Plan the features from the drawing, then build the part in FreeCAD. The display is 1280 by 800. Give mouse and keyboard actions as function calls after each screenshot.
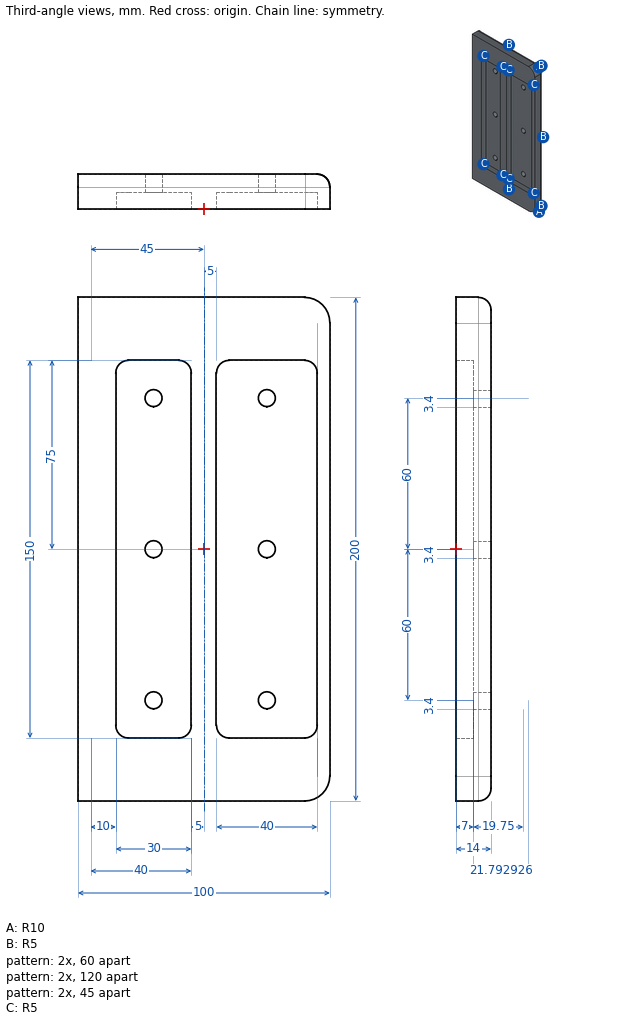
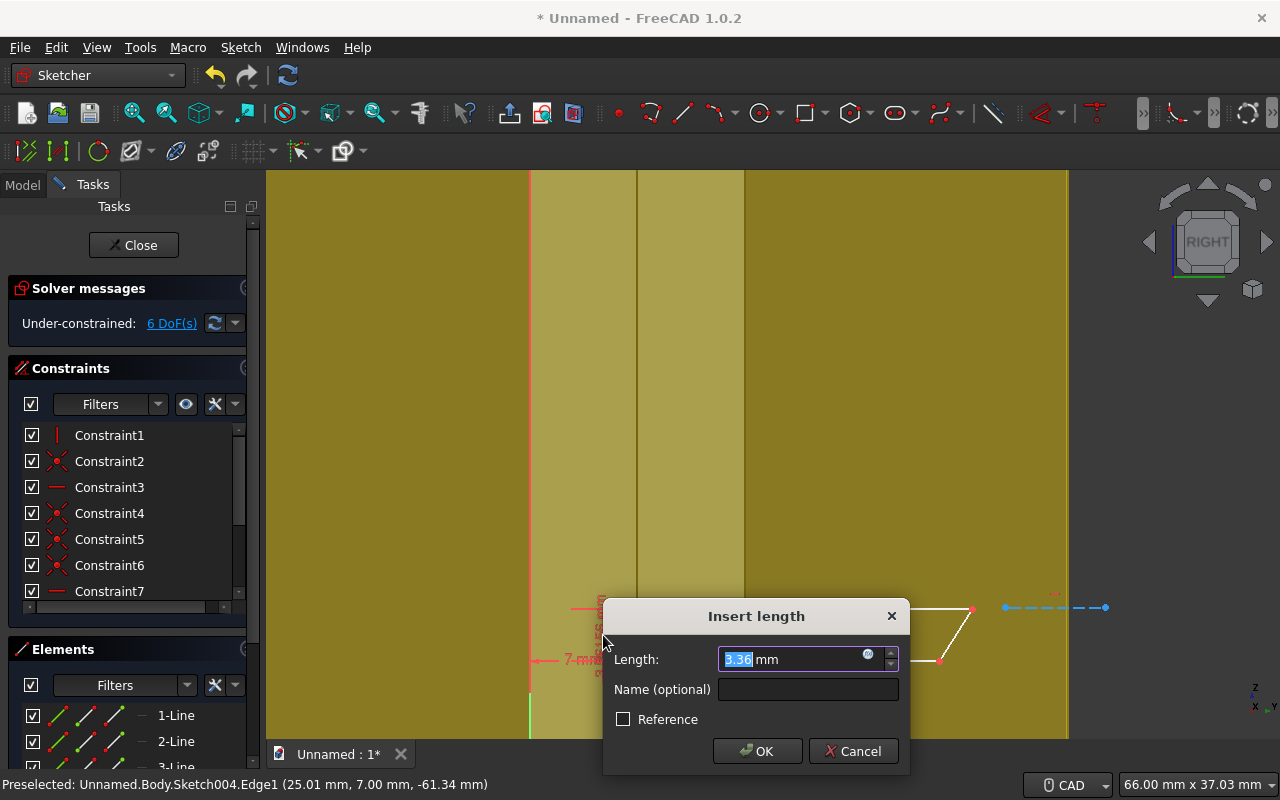
text(3.4)
key(Return)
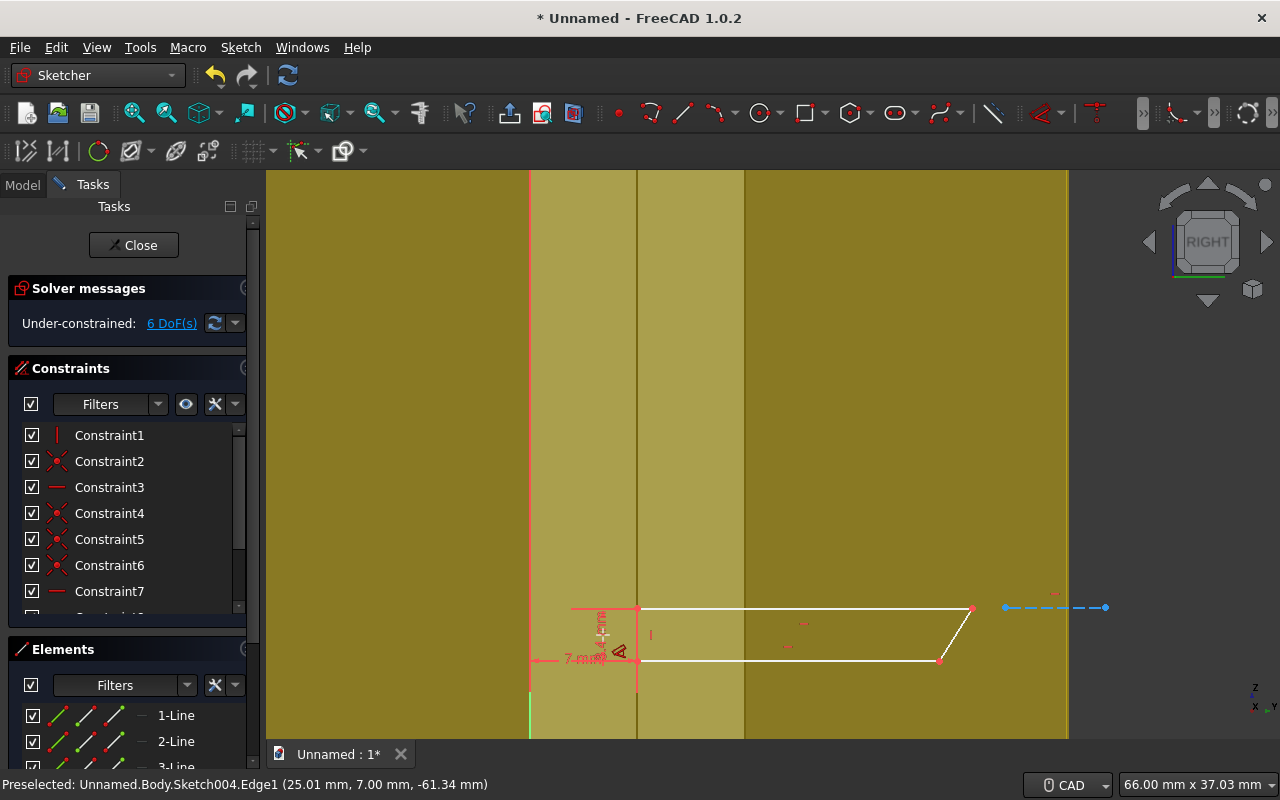
click(637, 609)
click(496, 403)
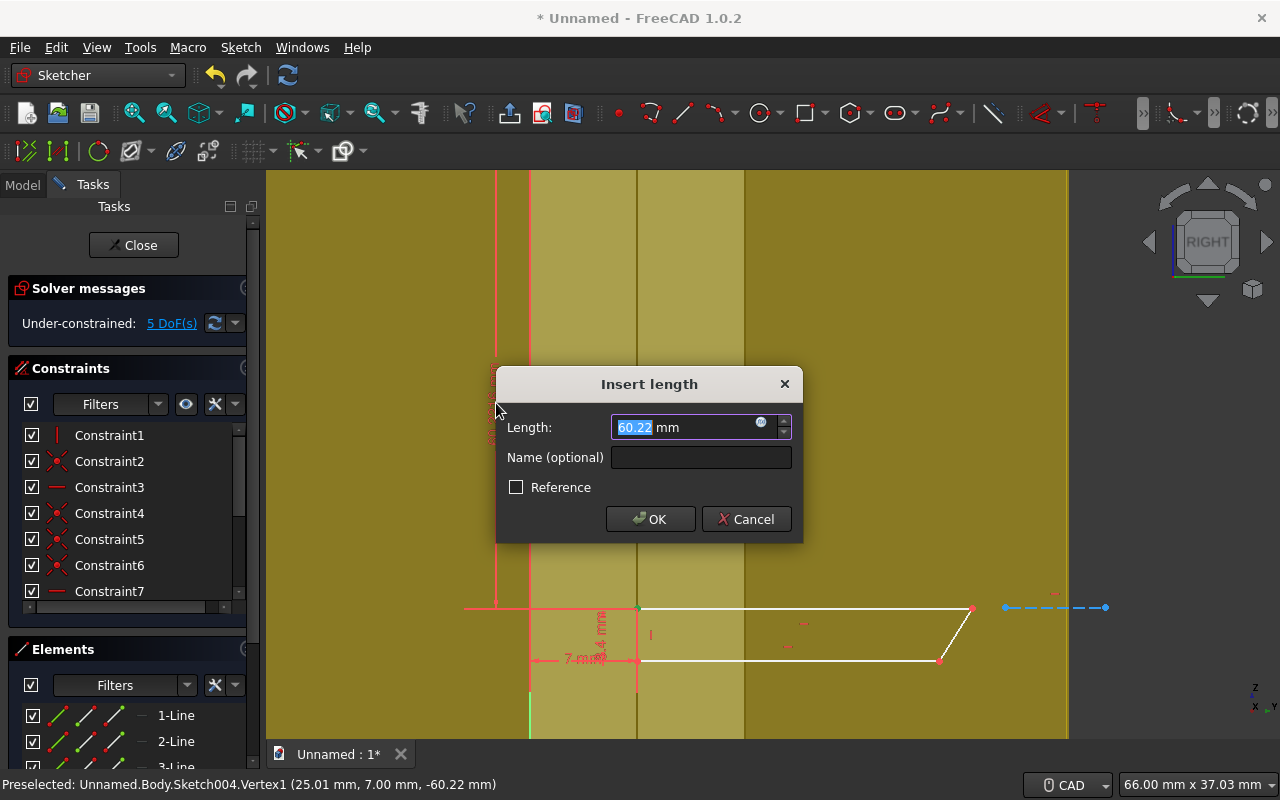
text(60)
key(Return)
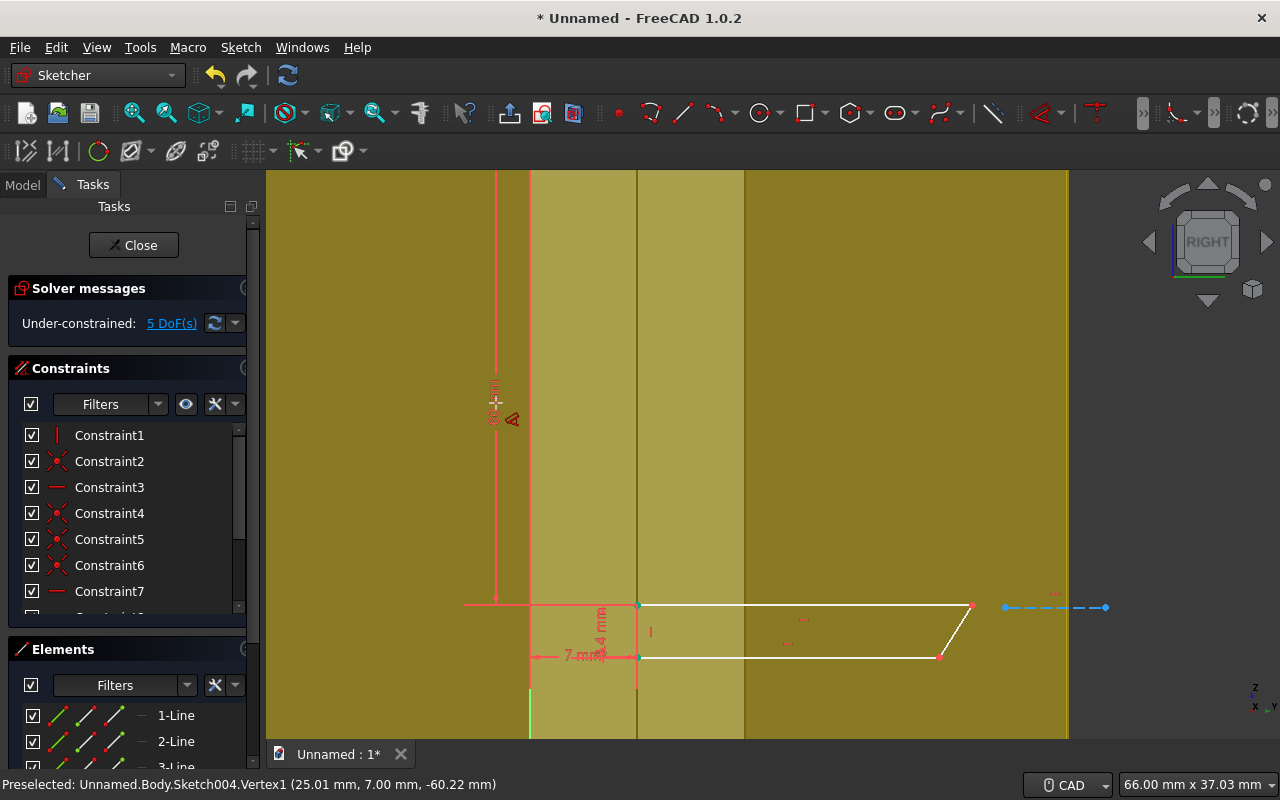
click(1005, 608)
click(496, 309)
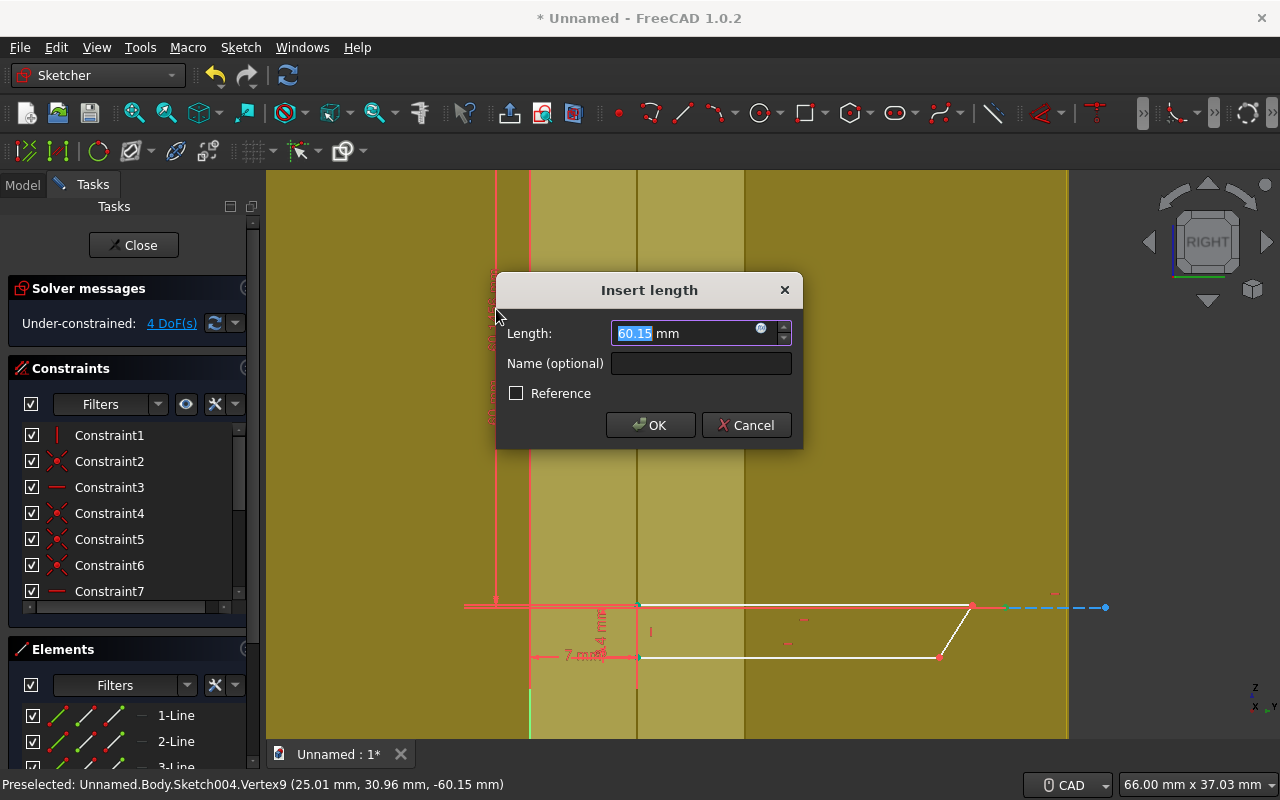
text(60)
key(Return)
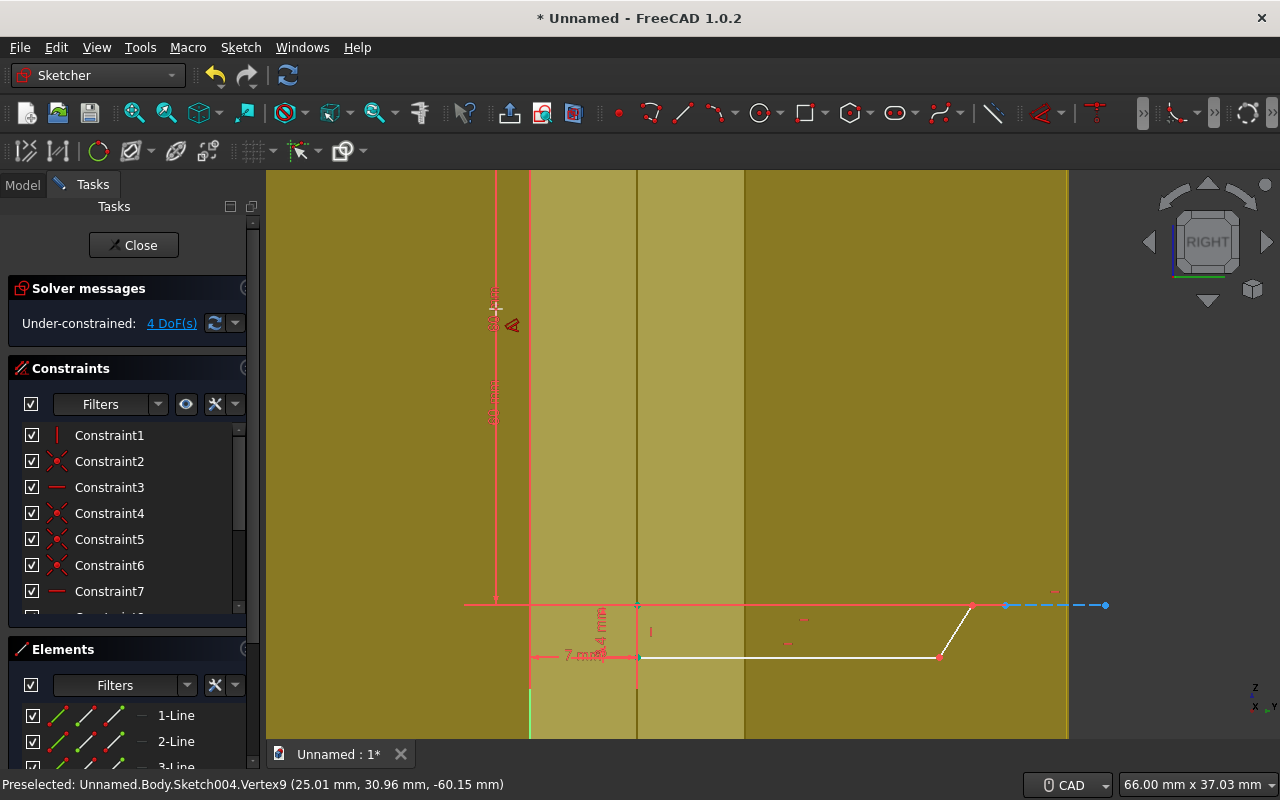
click(728, 658)
click(788, 692)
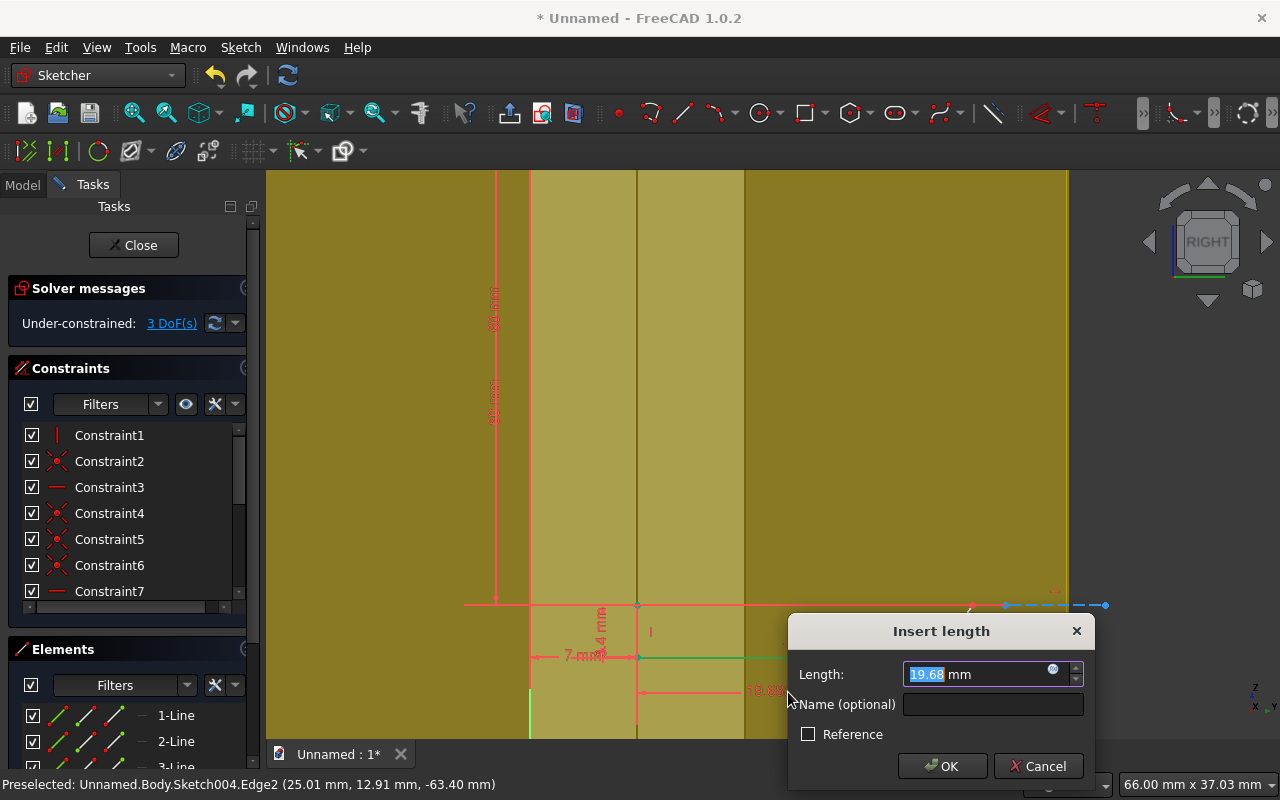
text(19.75)
key(Return)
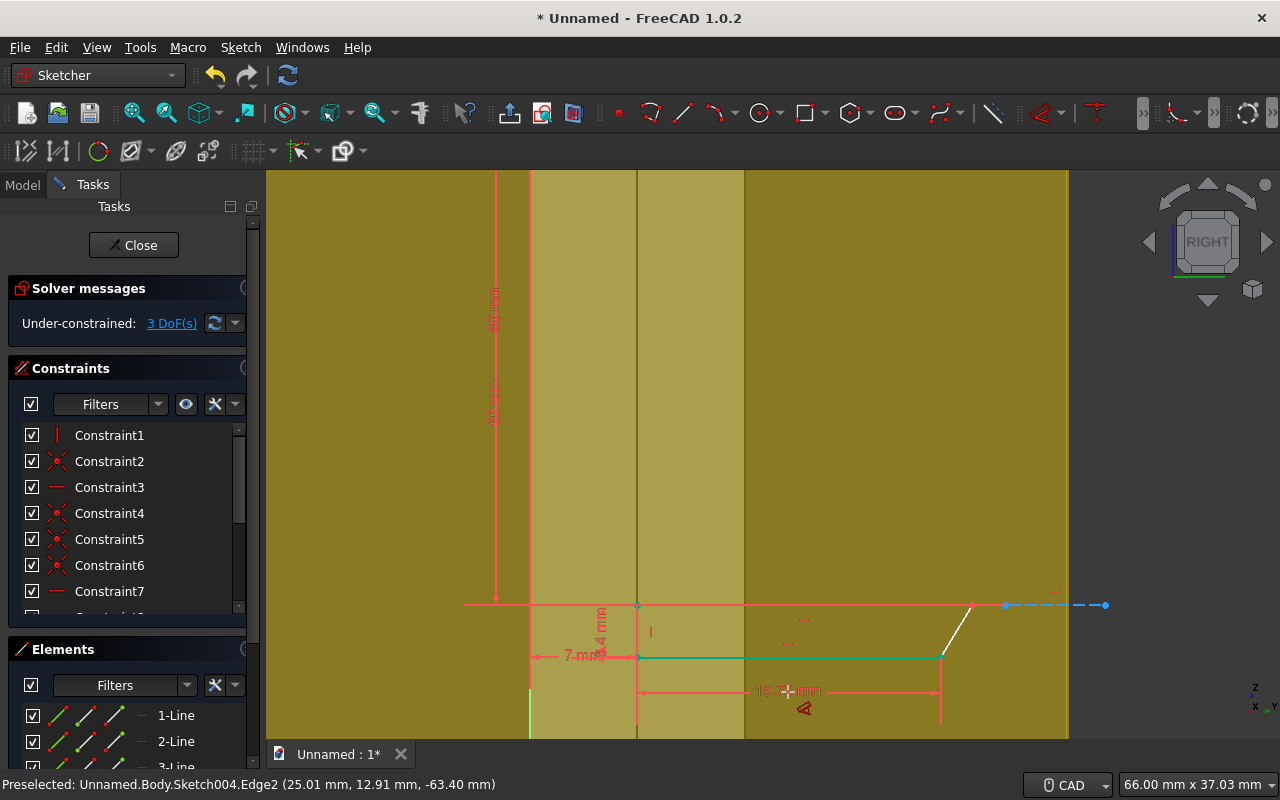
click(872, 605)
click(805, 639)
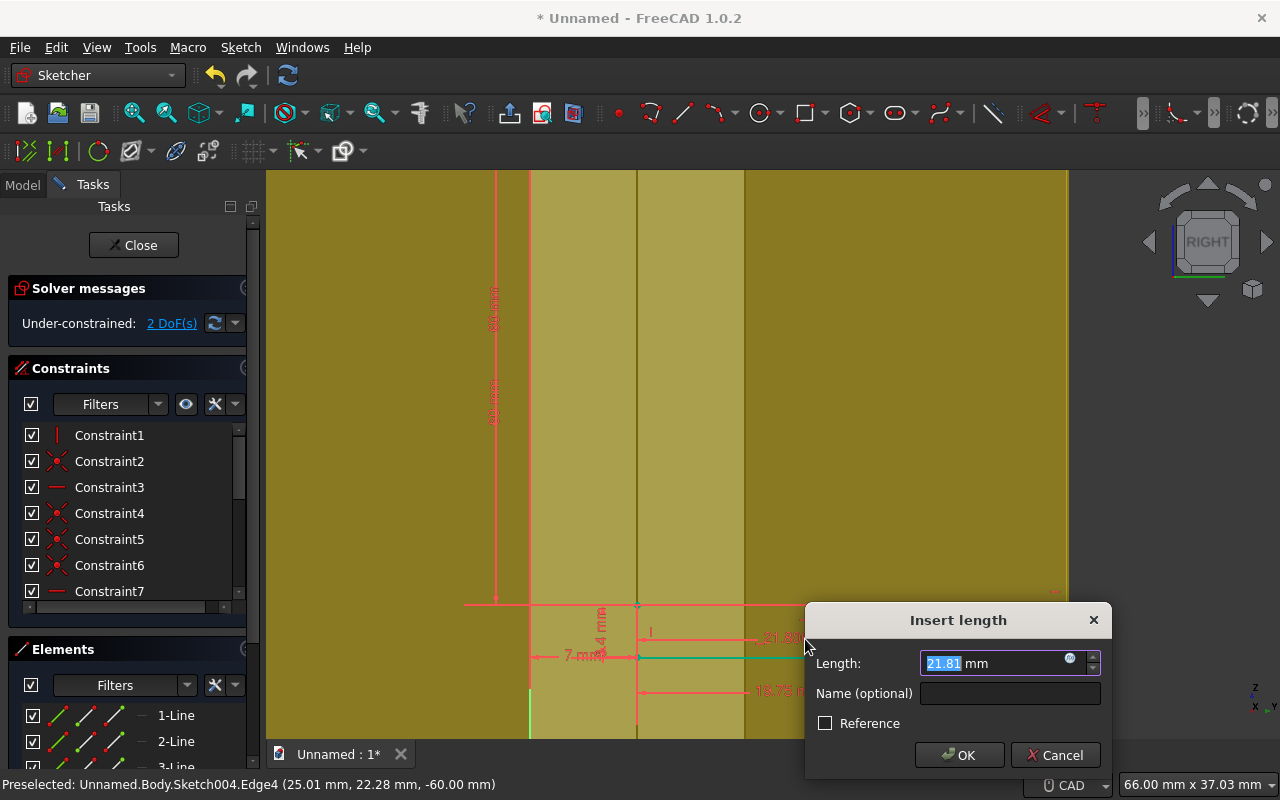
text(21.792926)
key(Return)
key(Escape)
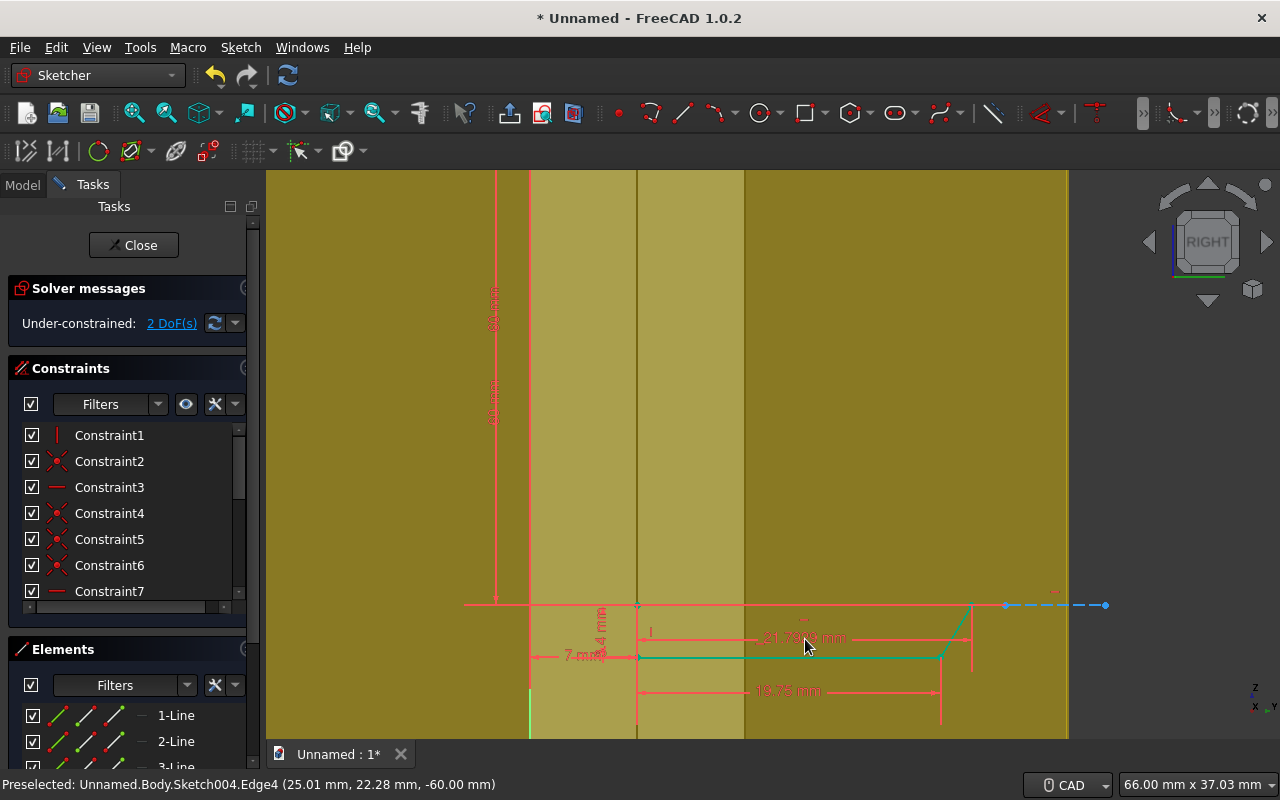
click(134, 245)